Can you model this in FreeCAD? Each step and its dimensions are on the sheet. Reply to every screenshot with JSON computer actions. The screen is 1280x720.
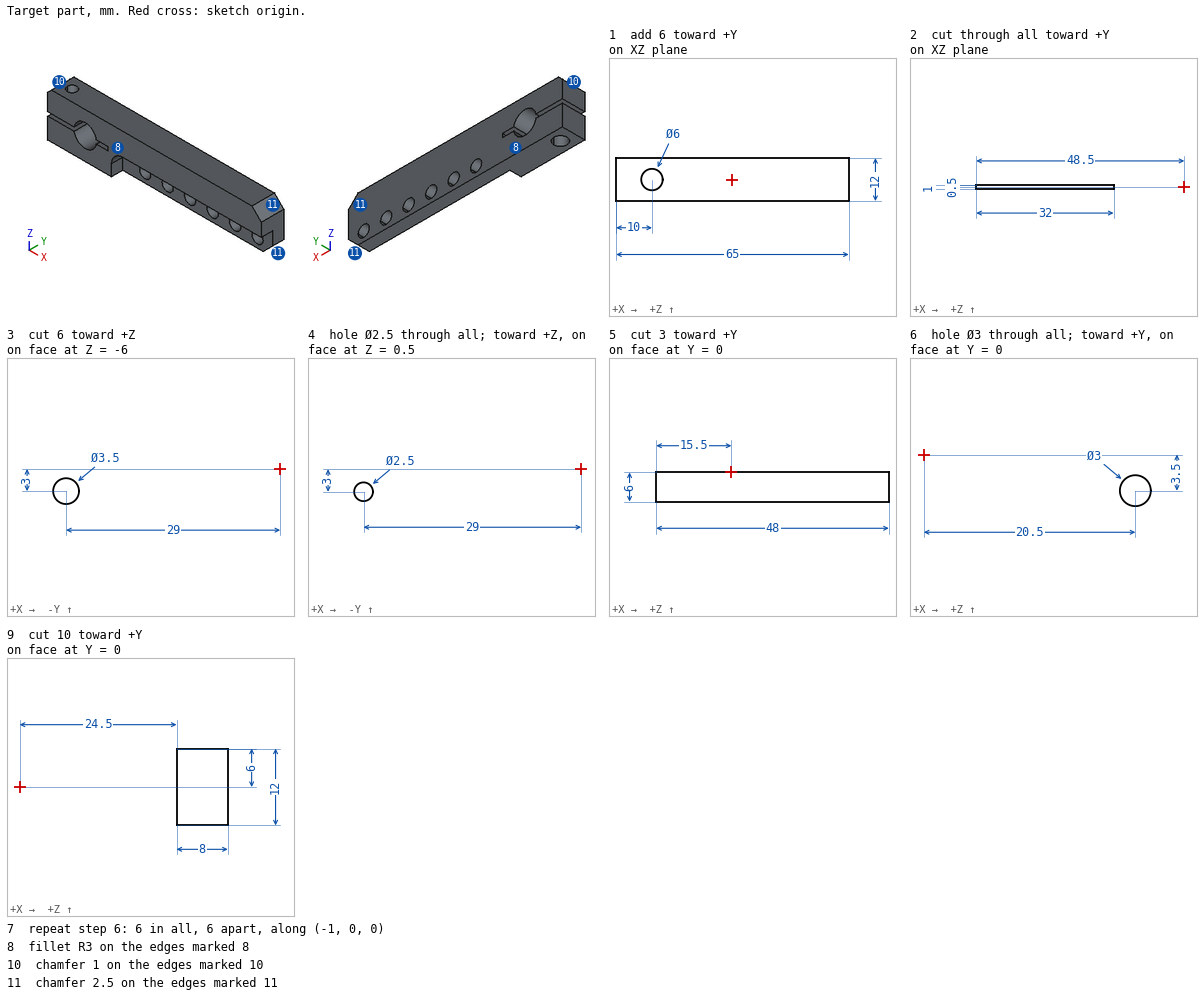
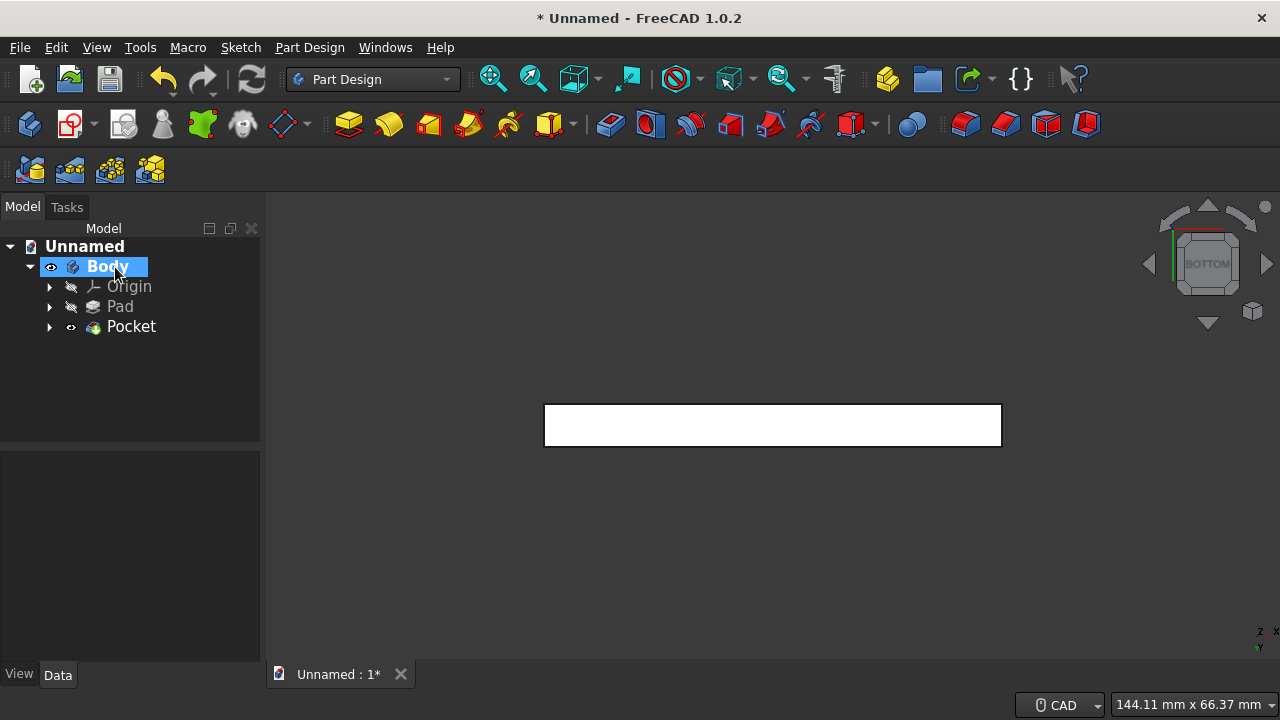
{"action": "left_click", "coordinate": [969, 424]}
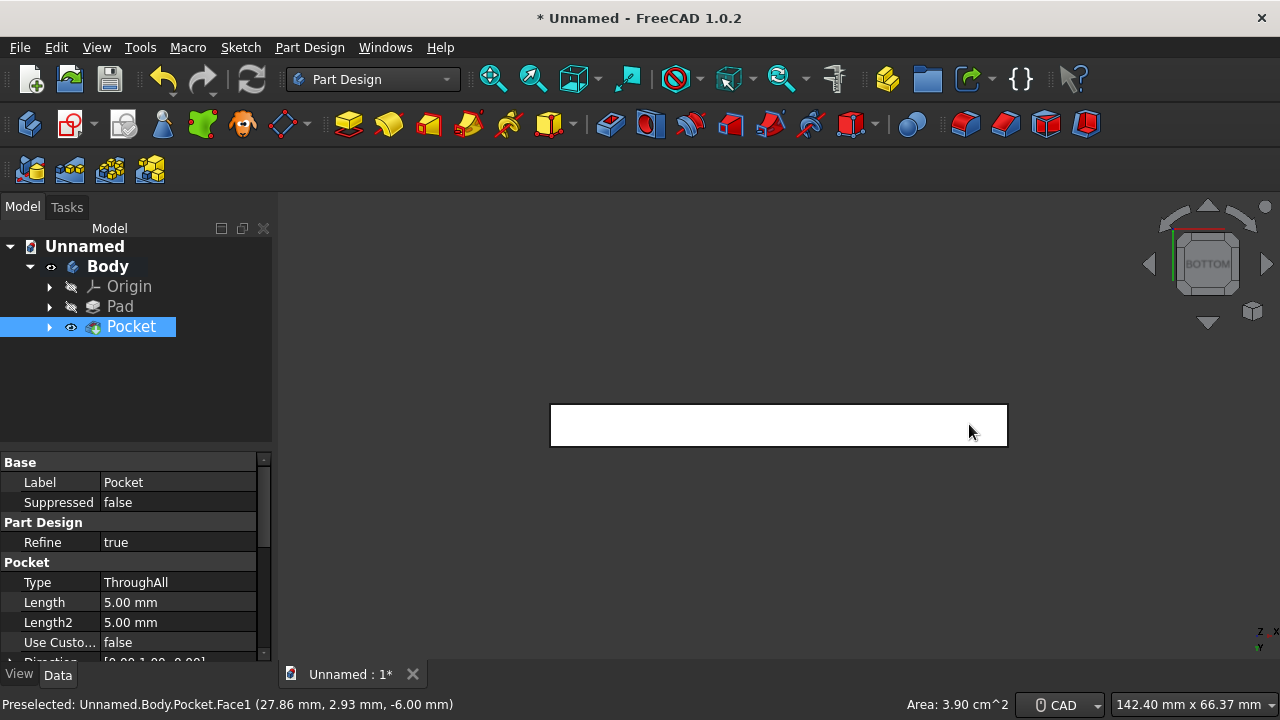
{"action": "left_click", "coordinate": [70, 124]}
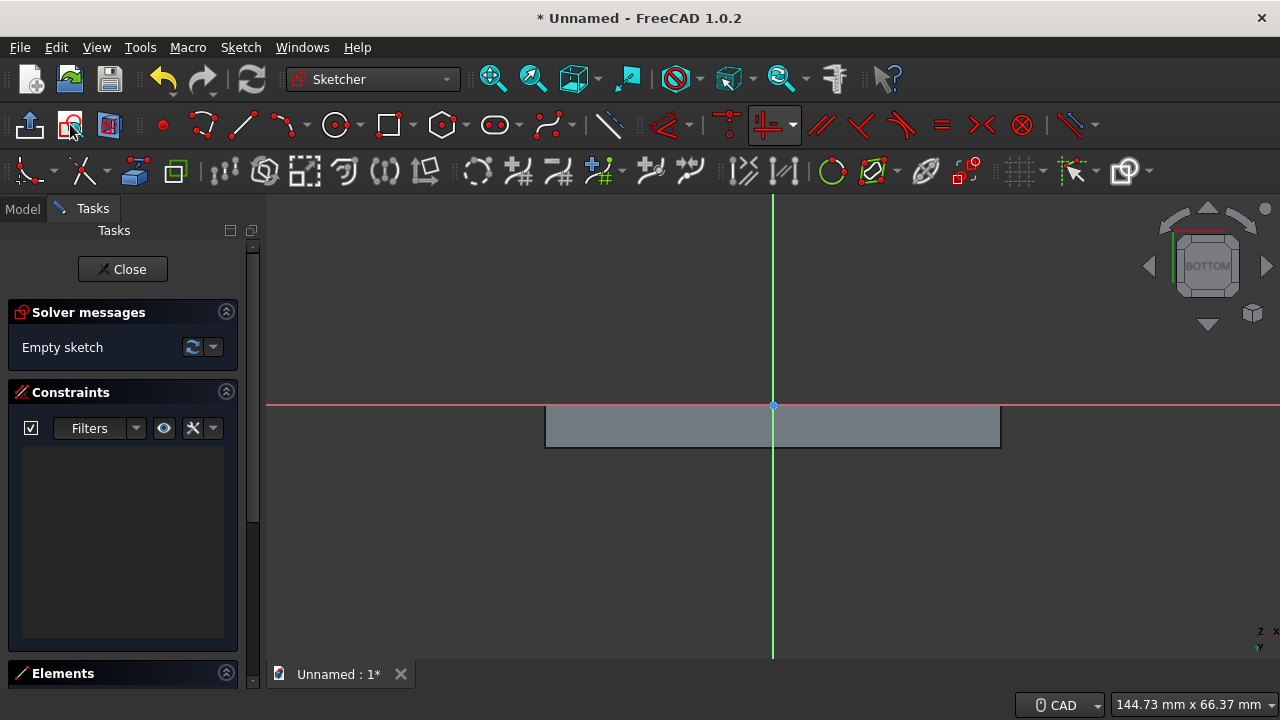
{"action": "scroll", "coordinate": [556, 426], "scroll_direction": "up", "scroll_amount": 12}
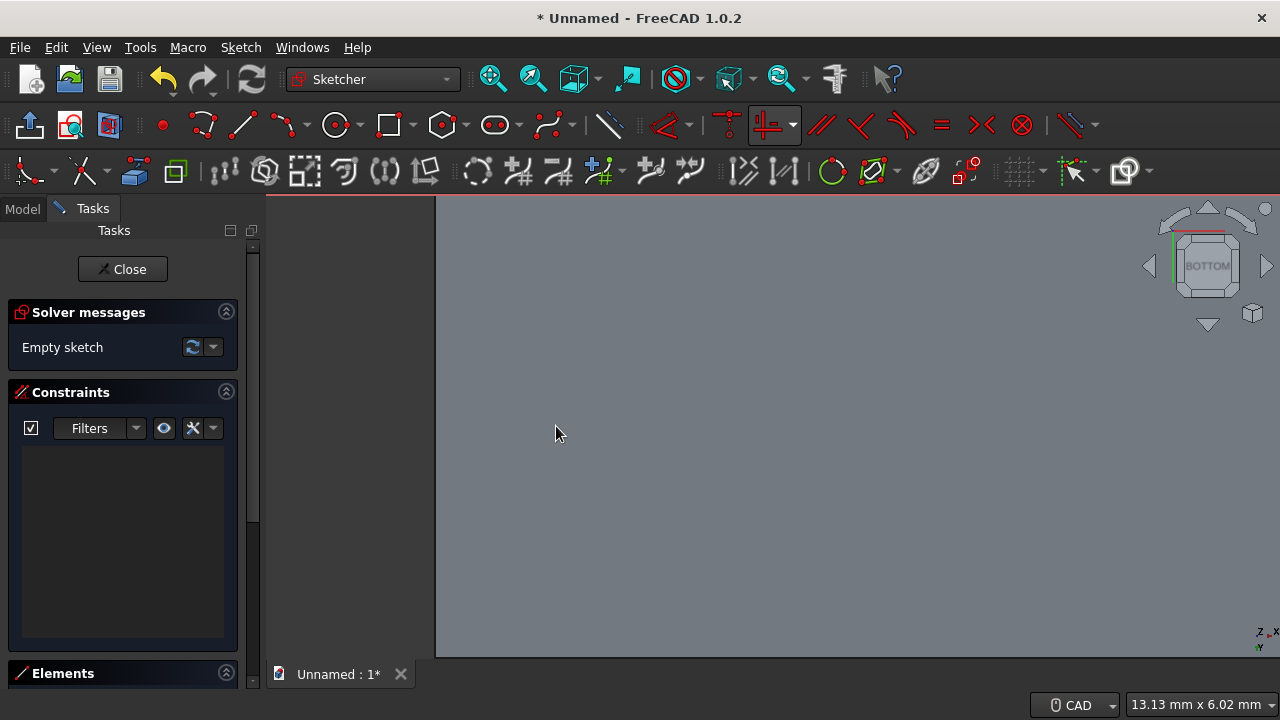
{"action": "key", "text": "g c"}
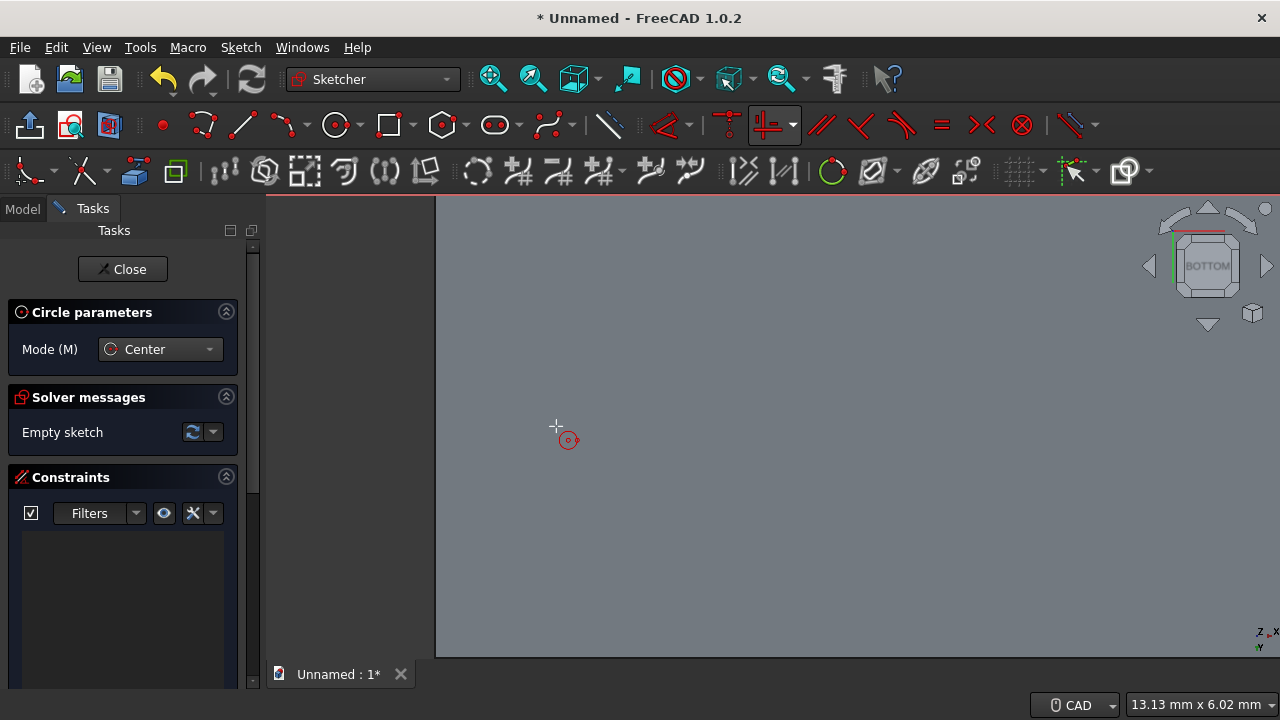
{"action": "left_click", "coordinate": [705, 426]}
{"action": "left_click", "coordinate": [801, 331]}
{"action": "key", "text": "Escape"}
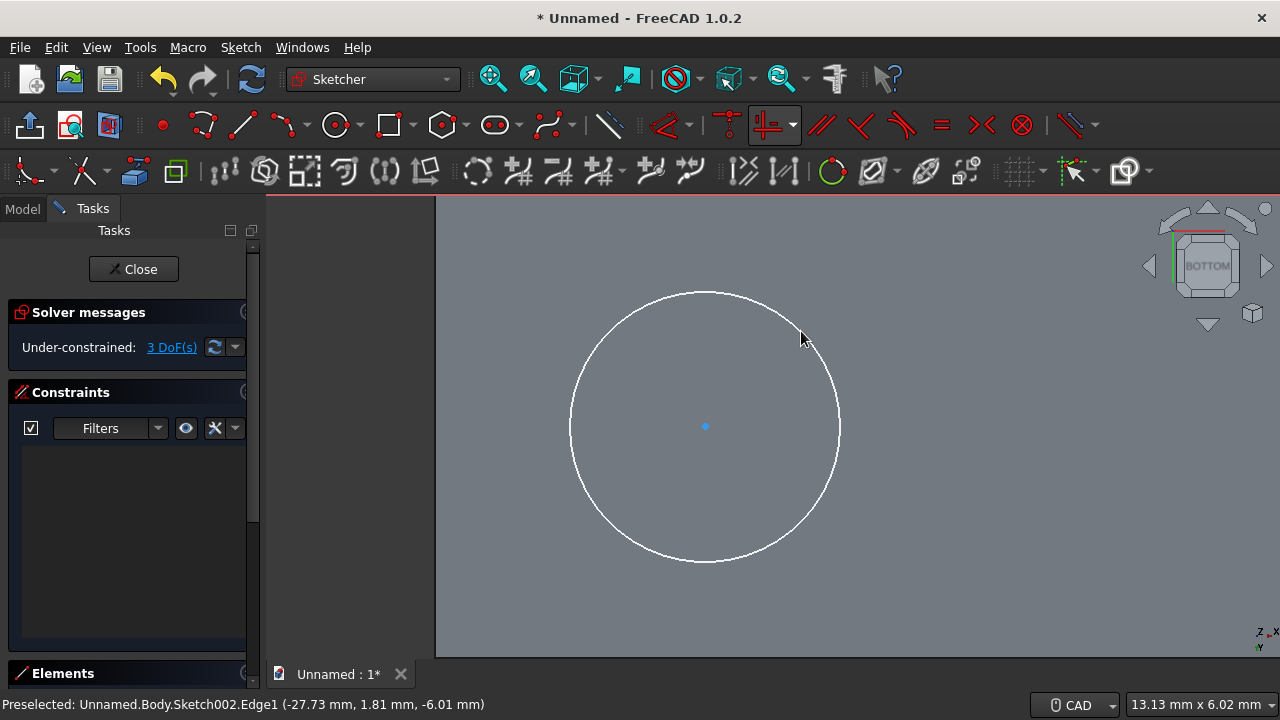
{"action": "key", "text": "d"}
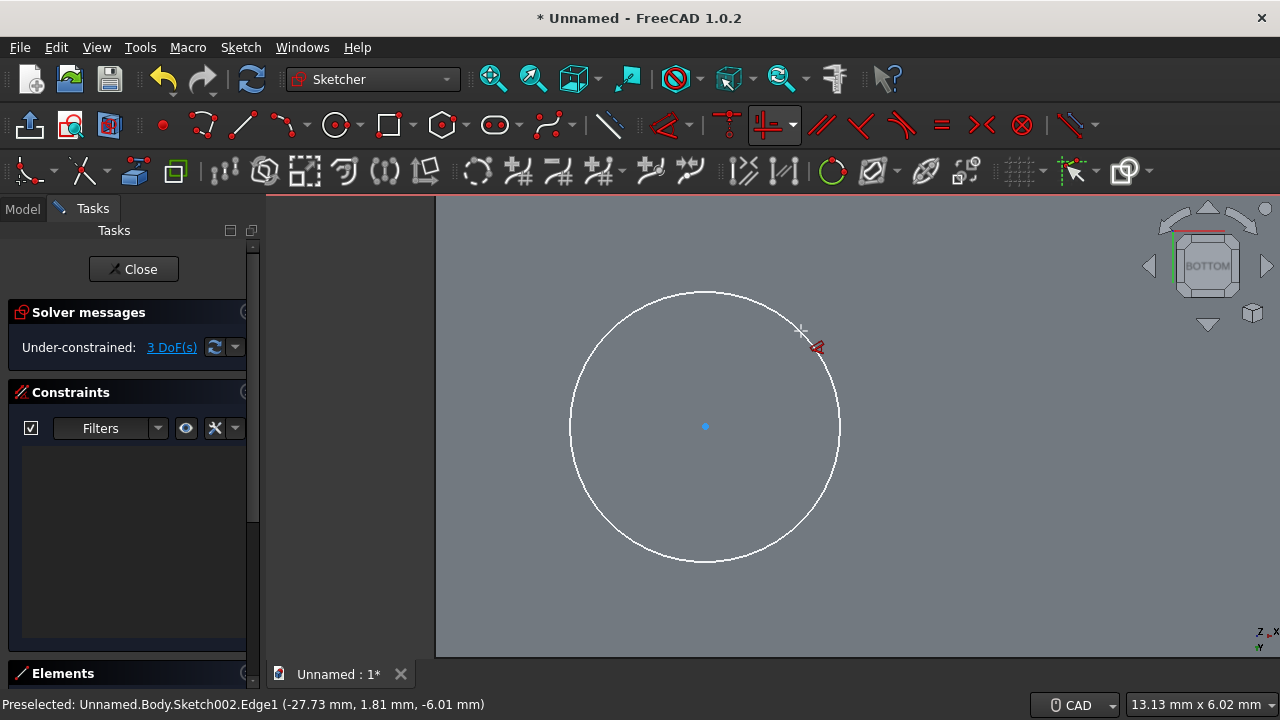
{"action": "left_click", "coordinate": [800, 331]}
{"action": "left_click", "coordinate": [823, 308]}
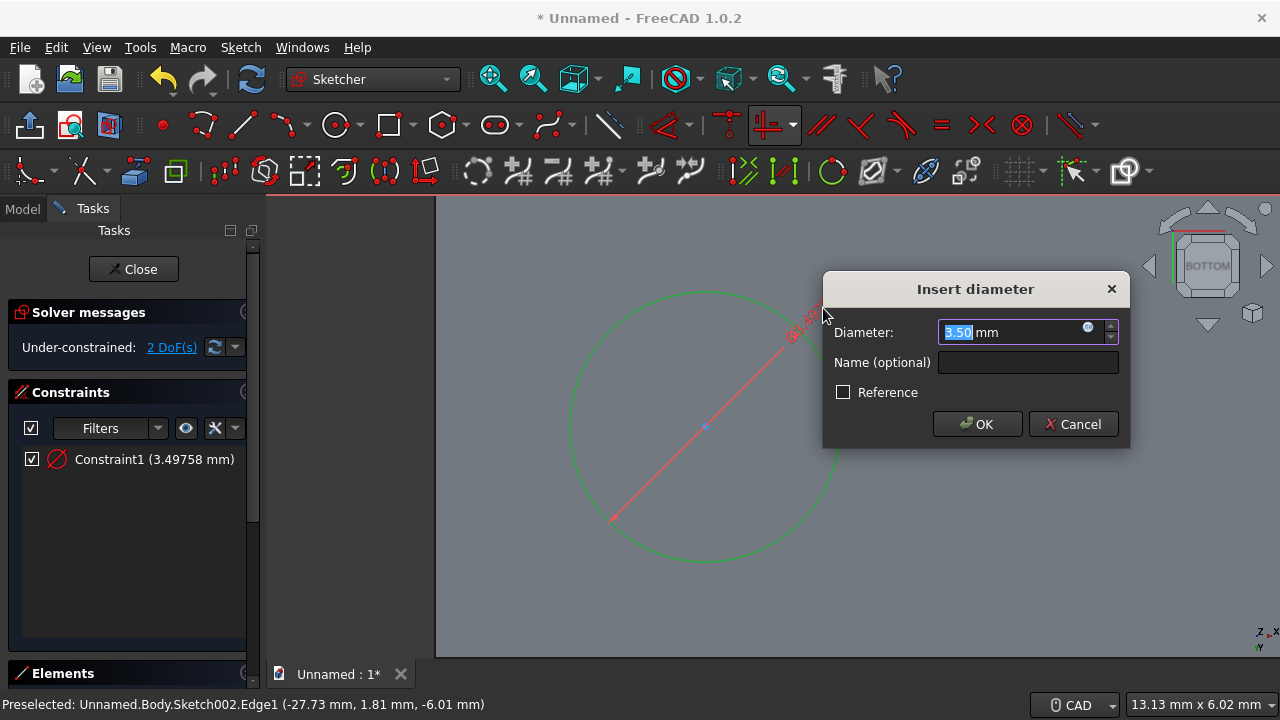
{"action": "type", "text": "3.5"}
{"action": "key", "text": "Return"}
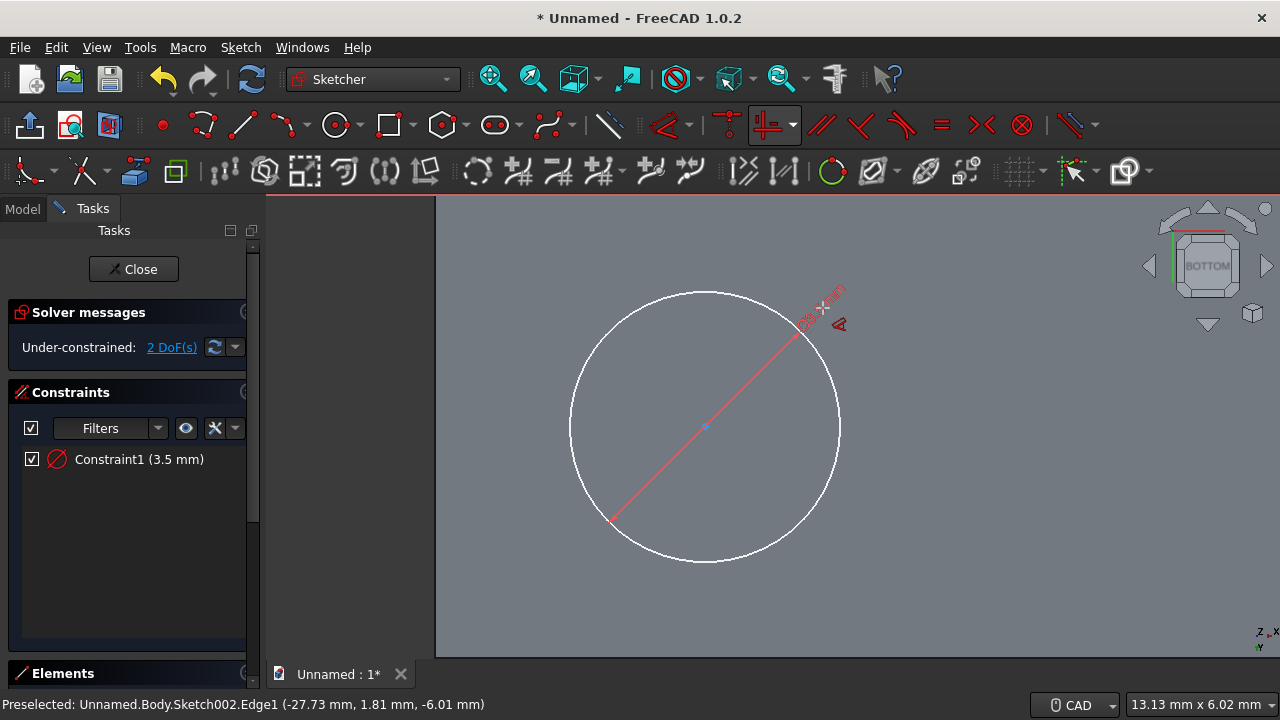
{"action": "left_click", "coordinate": [705, 427]}
{"action": "left_click", "coordinate": [671, 324]}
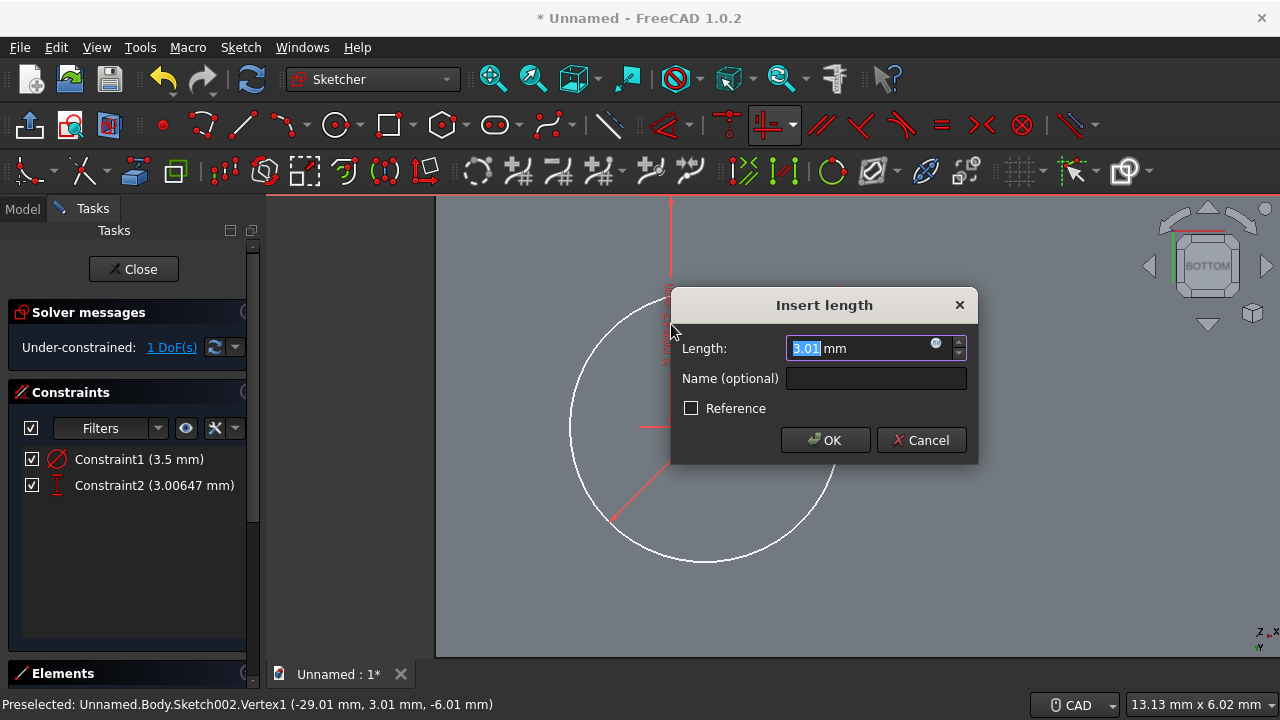
{"action": "type", "text": "3"}
{"action": "key", "text": "Return"}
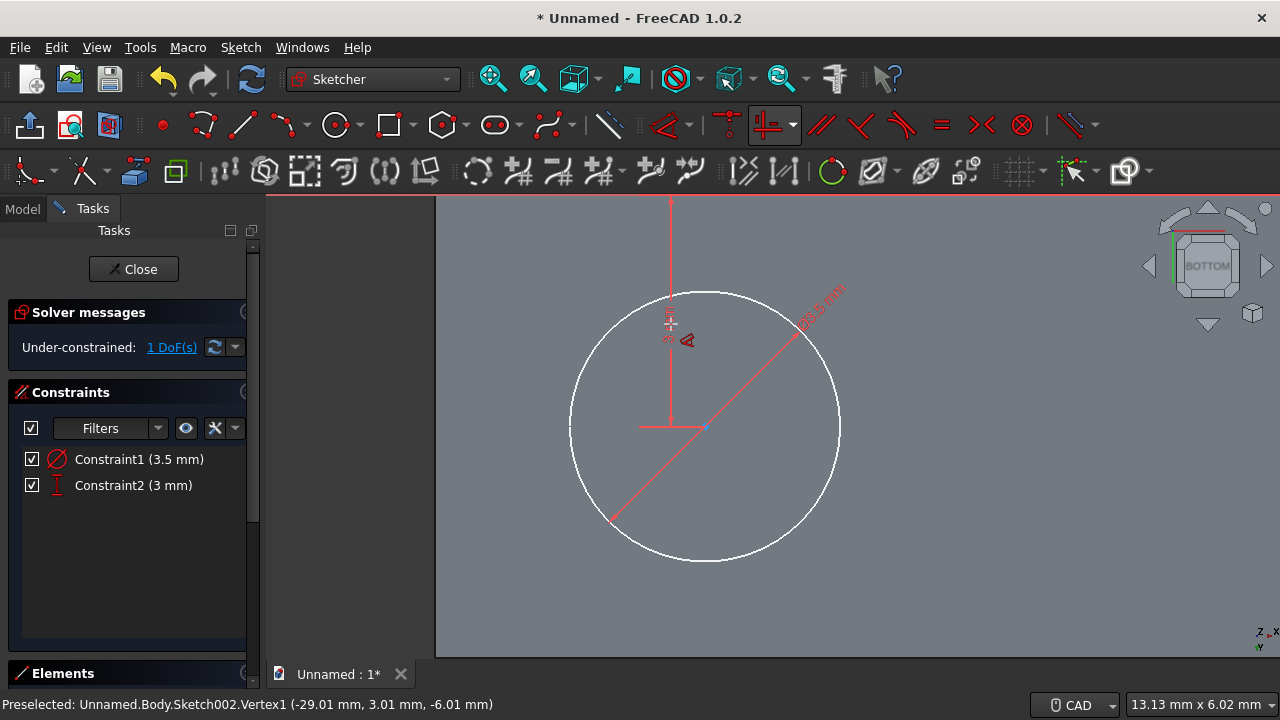
{"action": "left_click", "coordinate": [705, 426]}
{"action": "left_click", "coordinate": [910, 460]}